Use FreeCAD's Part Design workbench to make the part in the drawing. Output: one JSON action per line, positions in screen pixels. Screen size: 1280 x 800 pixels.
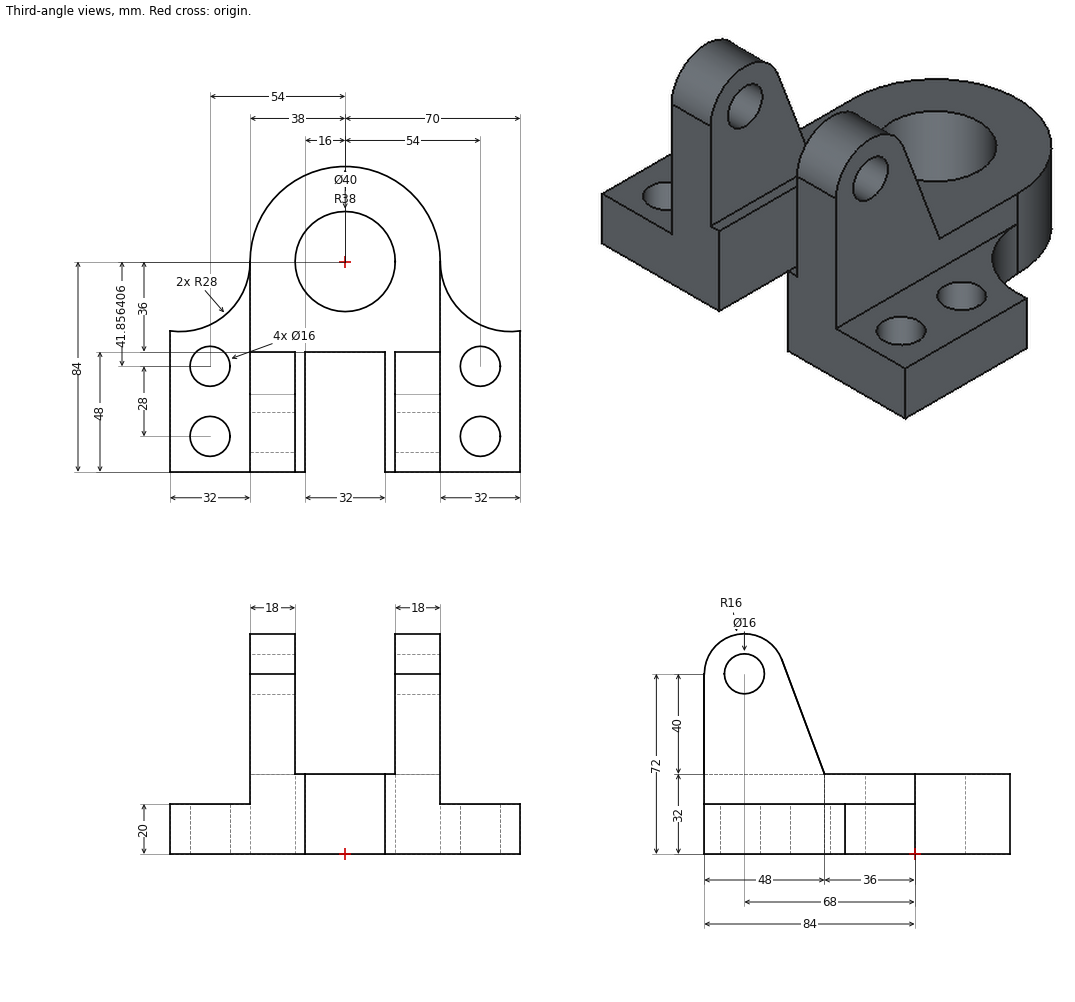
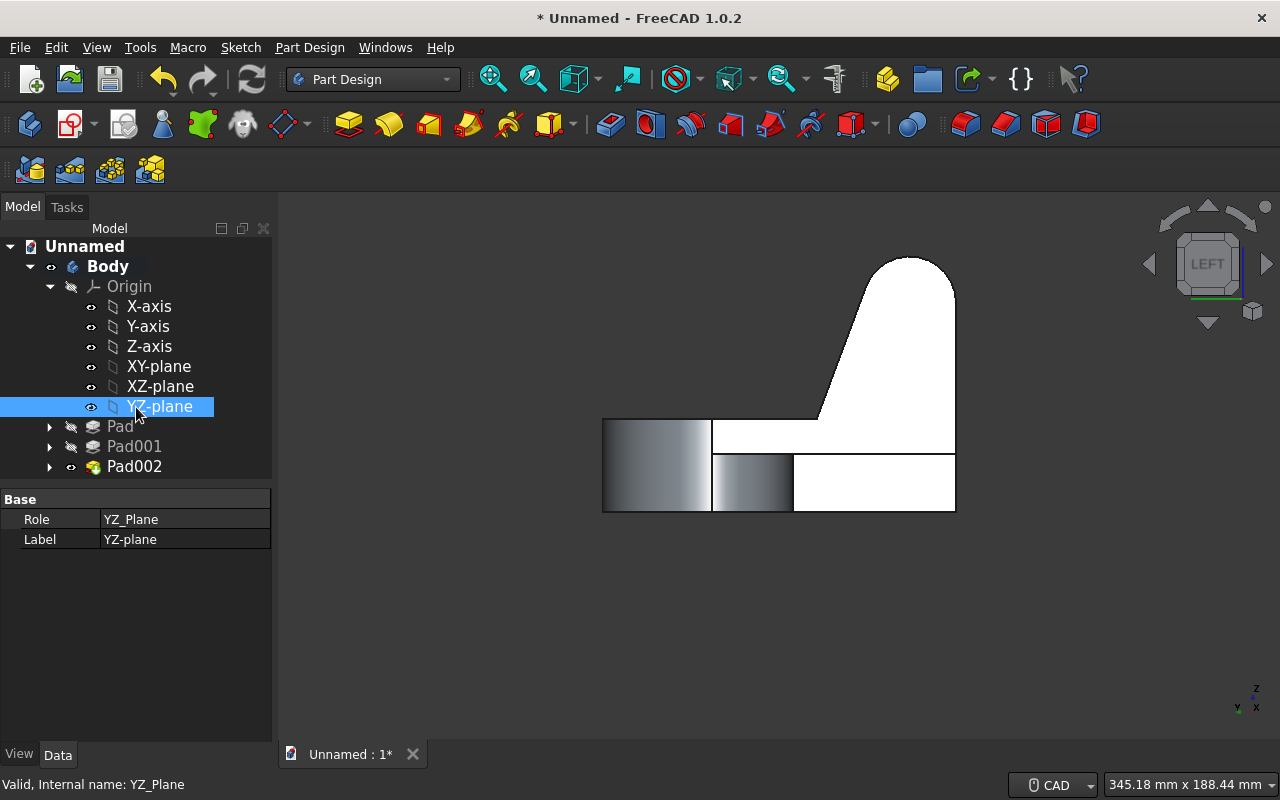
{"action": "left_click", "coordinate": [284, 124]}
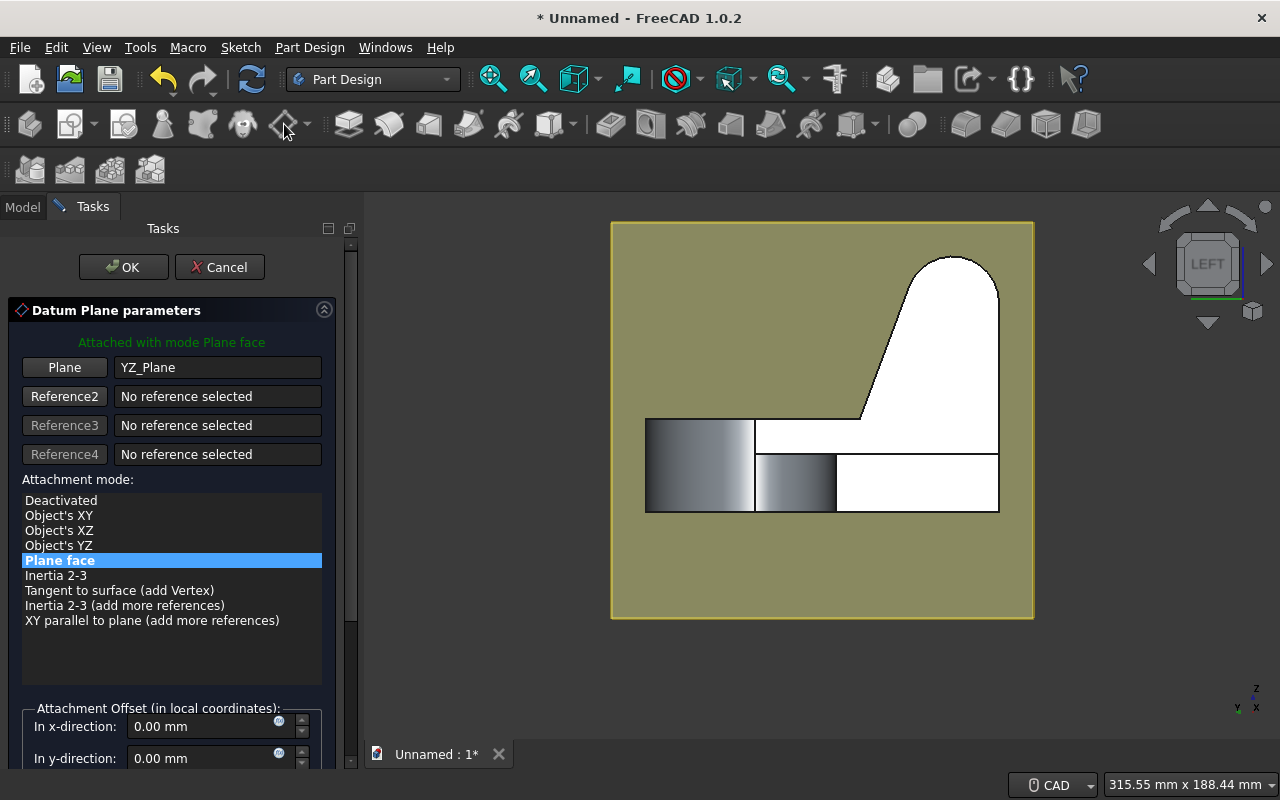
{"action": "scroll", "coordinate": [351, 503], "scroll_direction": "down", "scroll_amount": 2}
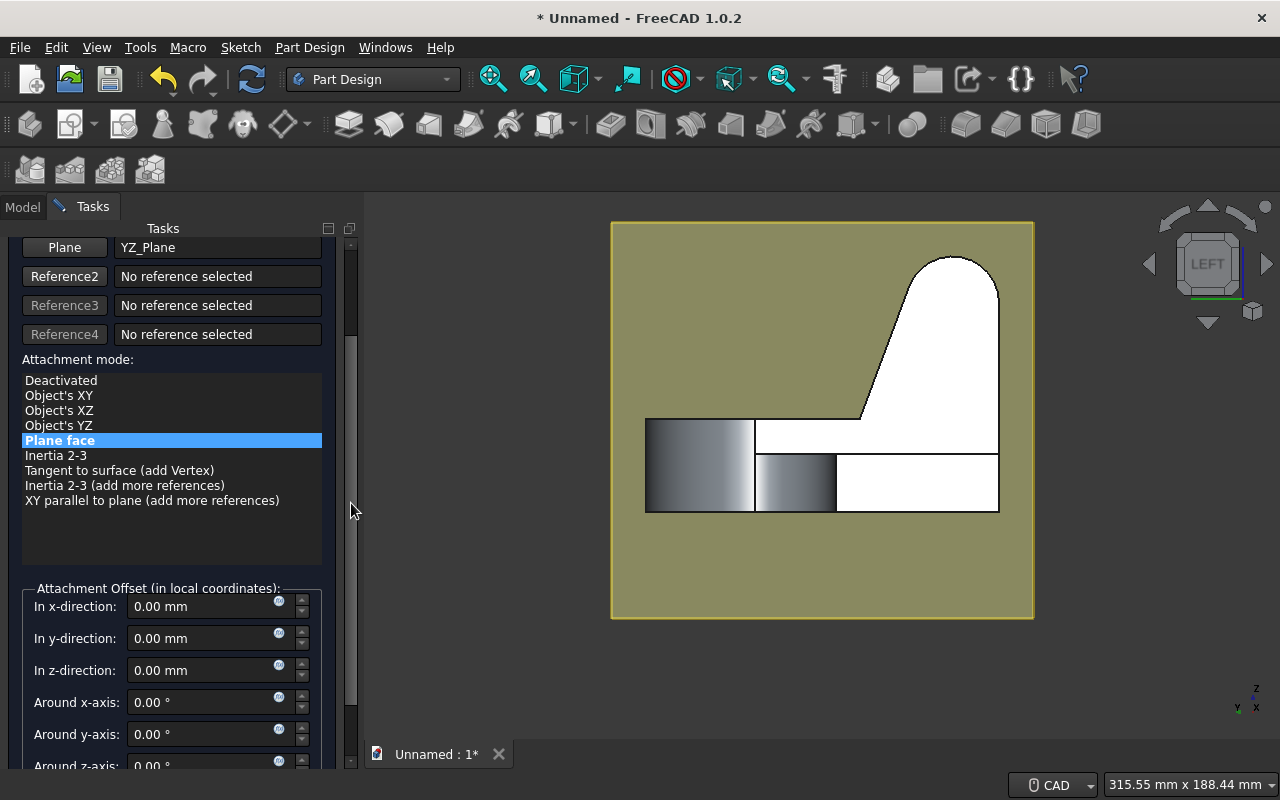
{"action": "triple_click", "coordinate": [210, 670]}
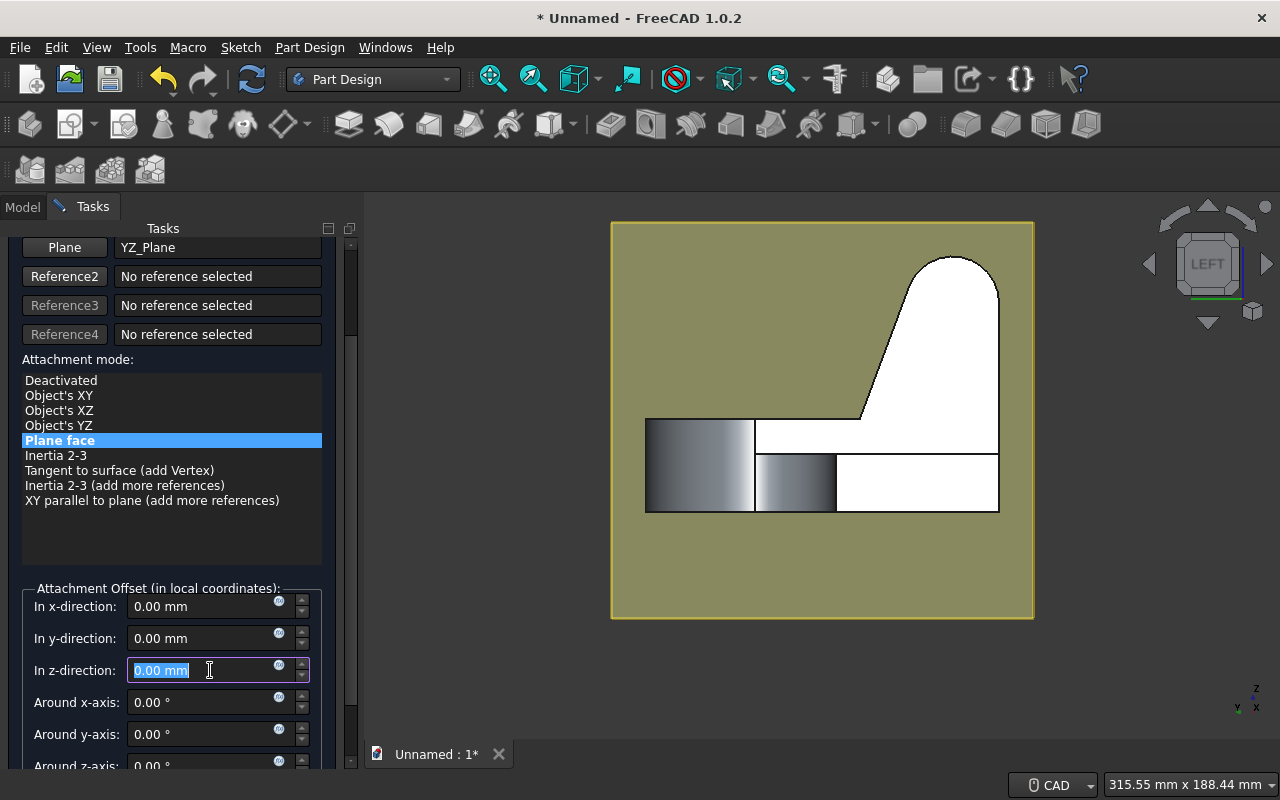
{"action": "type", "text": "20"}
{"action": "key", "text": "Tab"}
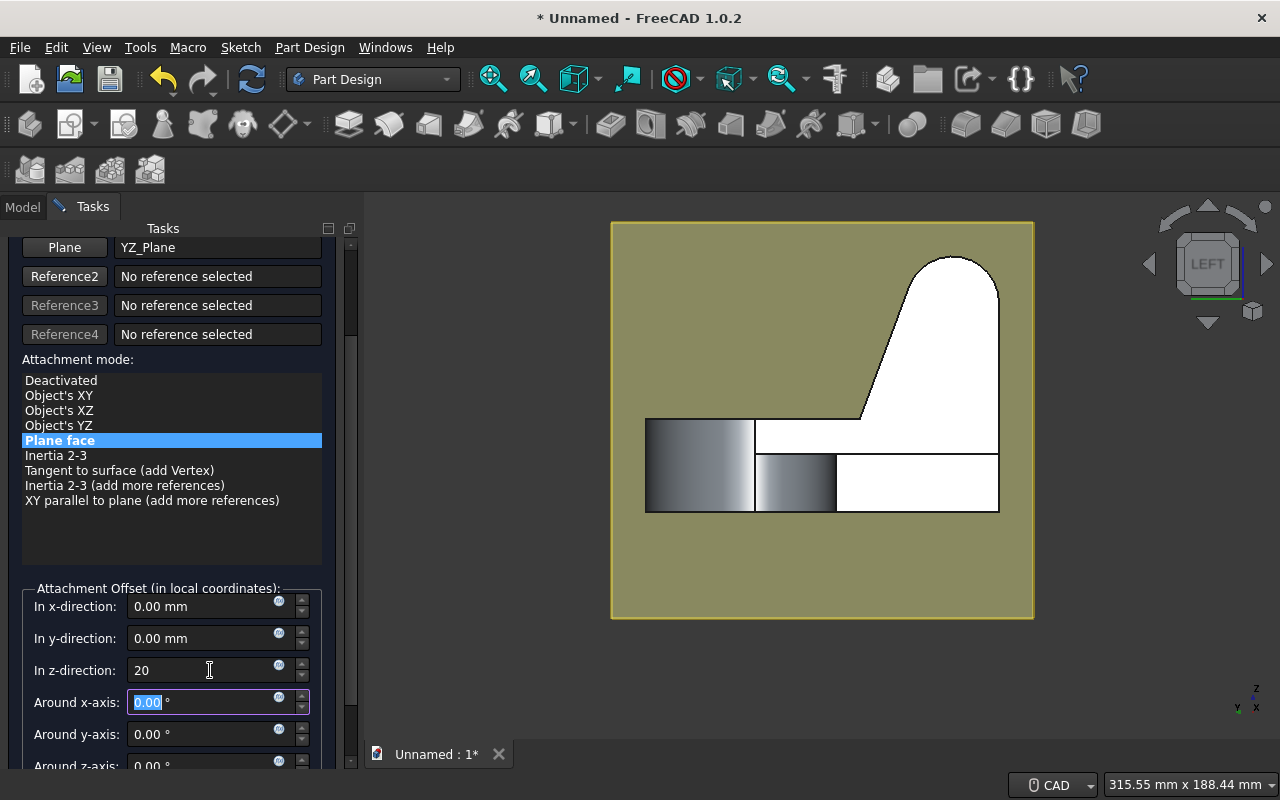
{"action": "scroll", "coordinate": [351, 503], "scroll_direction": "up", "scroll_amount": 3}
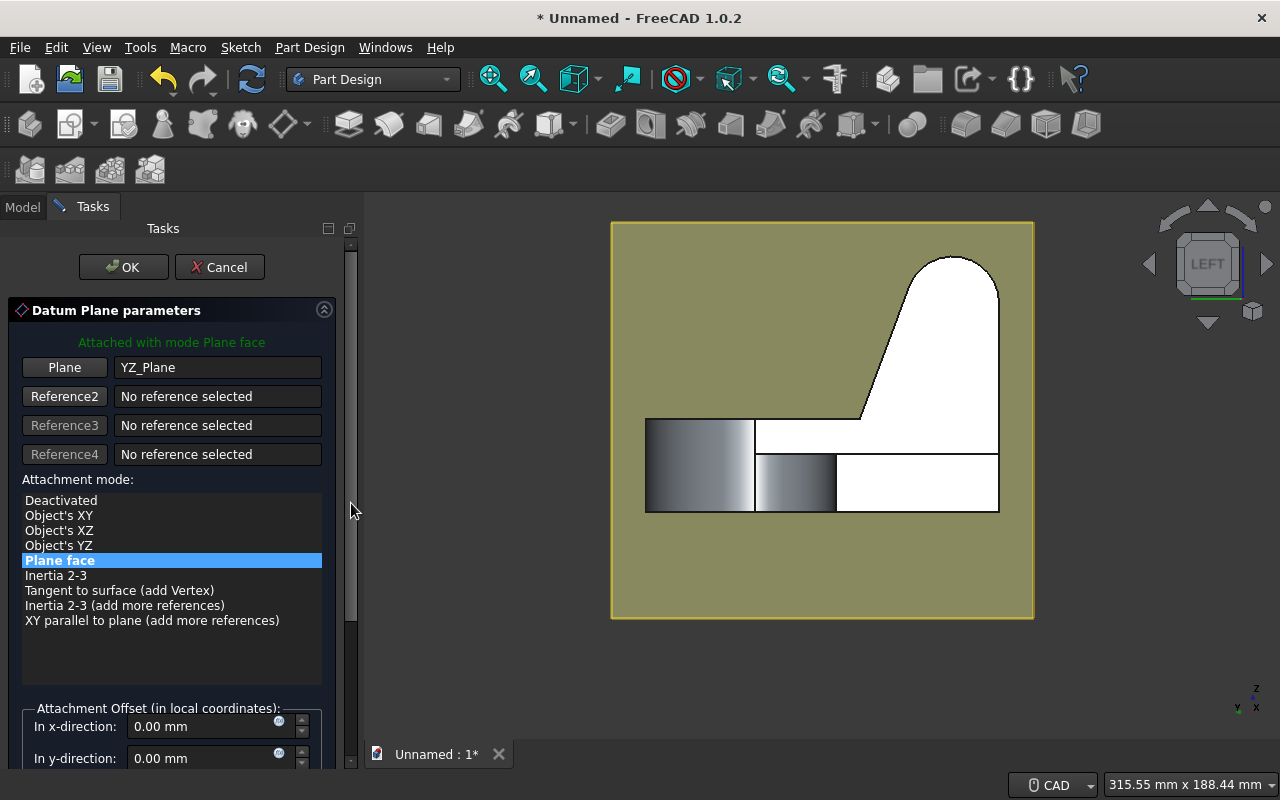
{"action": "left_click", "coordinate": [124, 267]}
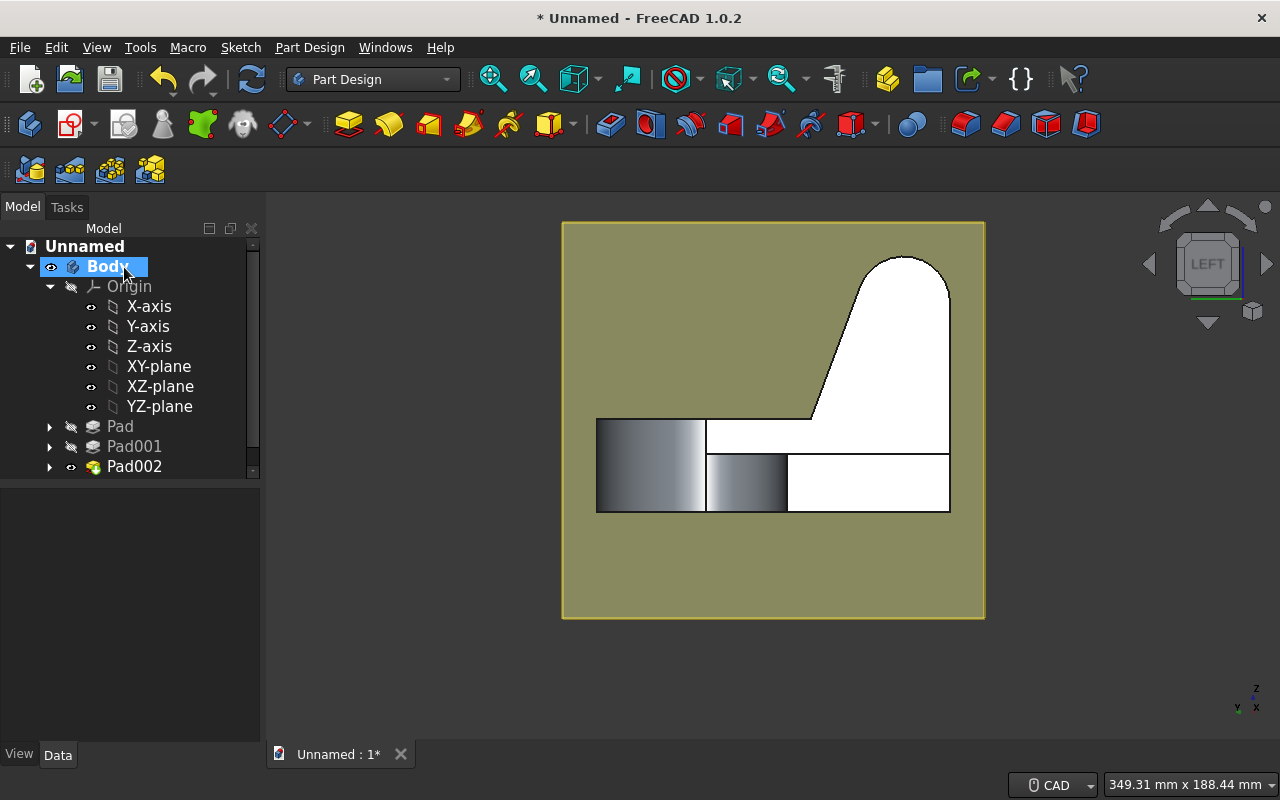
{"action": "scroll", "coordinate": [100, 362], "scroll_direction": "down", "scroll_amount": 3}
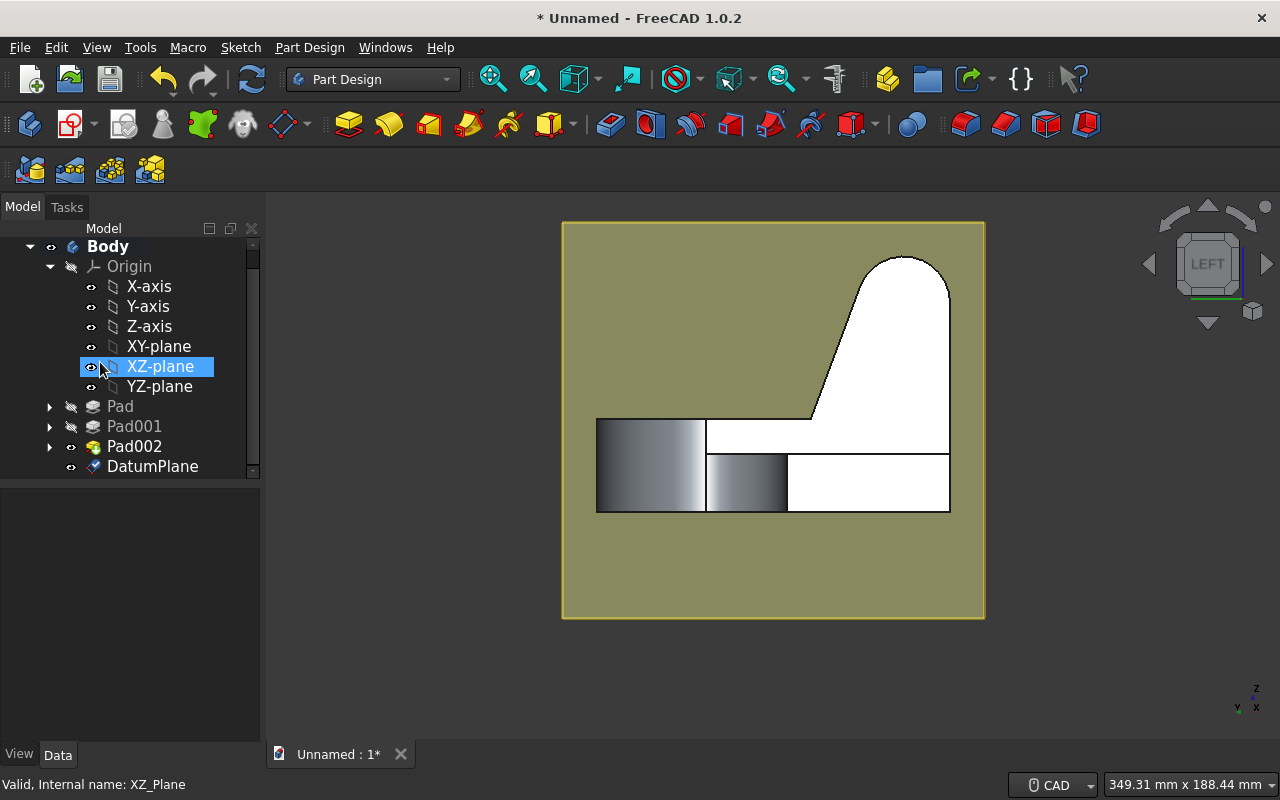
{"action": "left_click", "coordinate": [116, 467]}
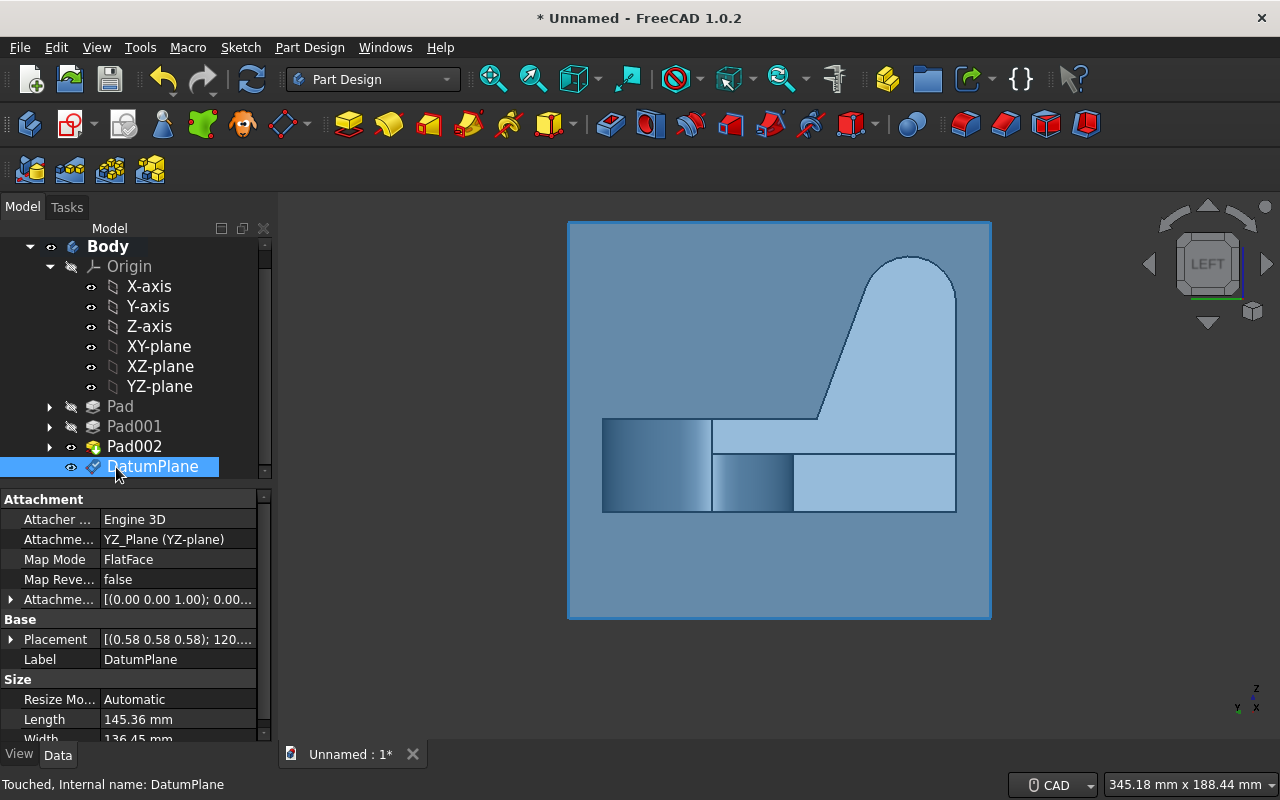
{"action": "left_click", "coordinate": [70, 124]}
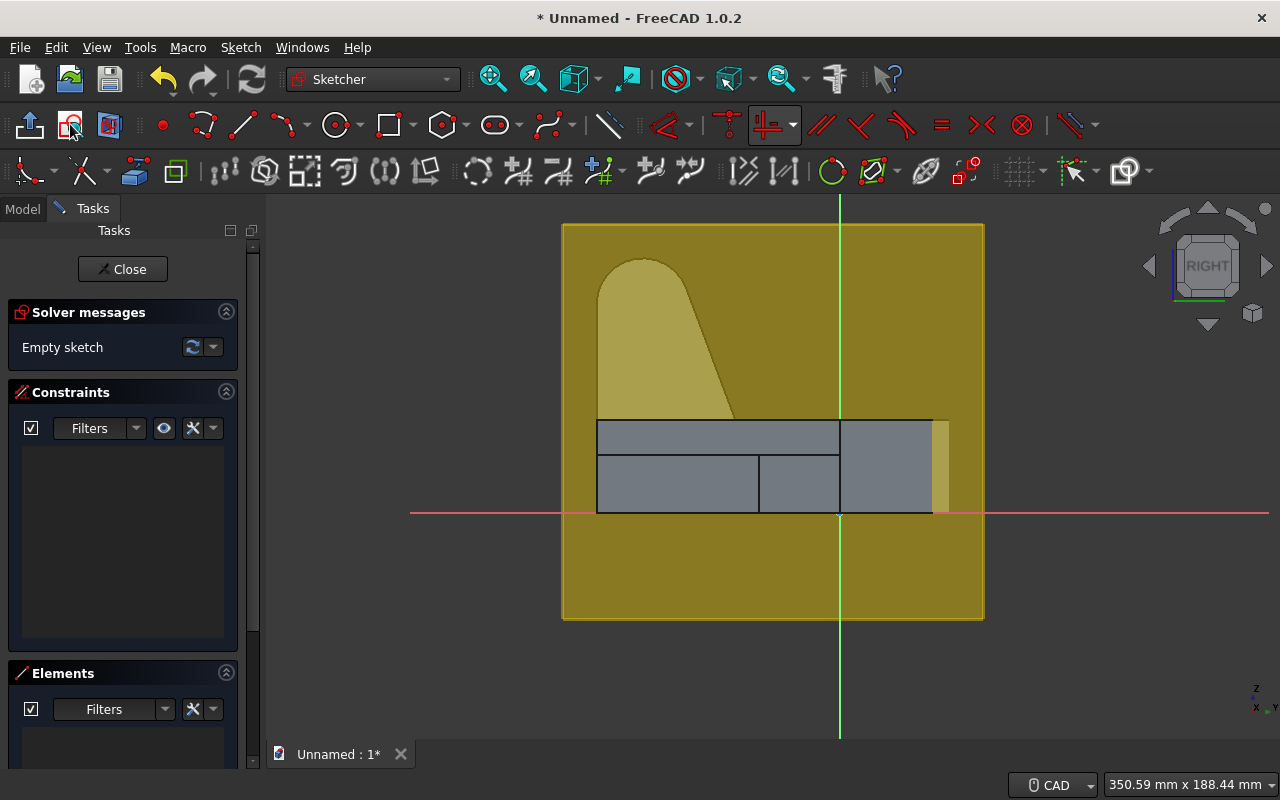
{"action": "left_click", "coordinate": [110, 126]}